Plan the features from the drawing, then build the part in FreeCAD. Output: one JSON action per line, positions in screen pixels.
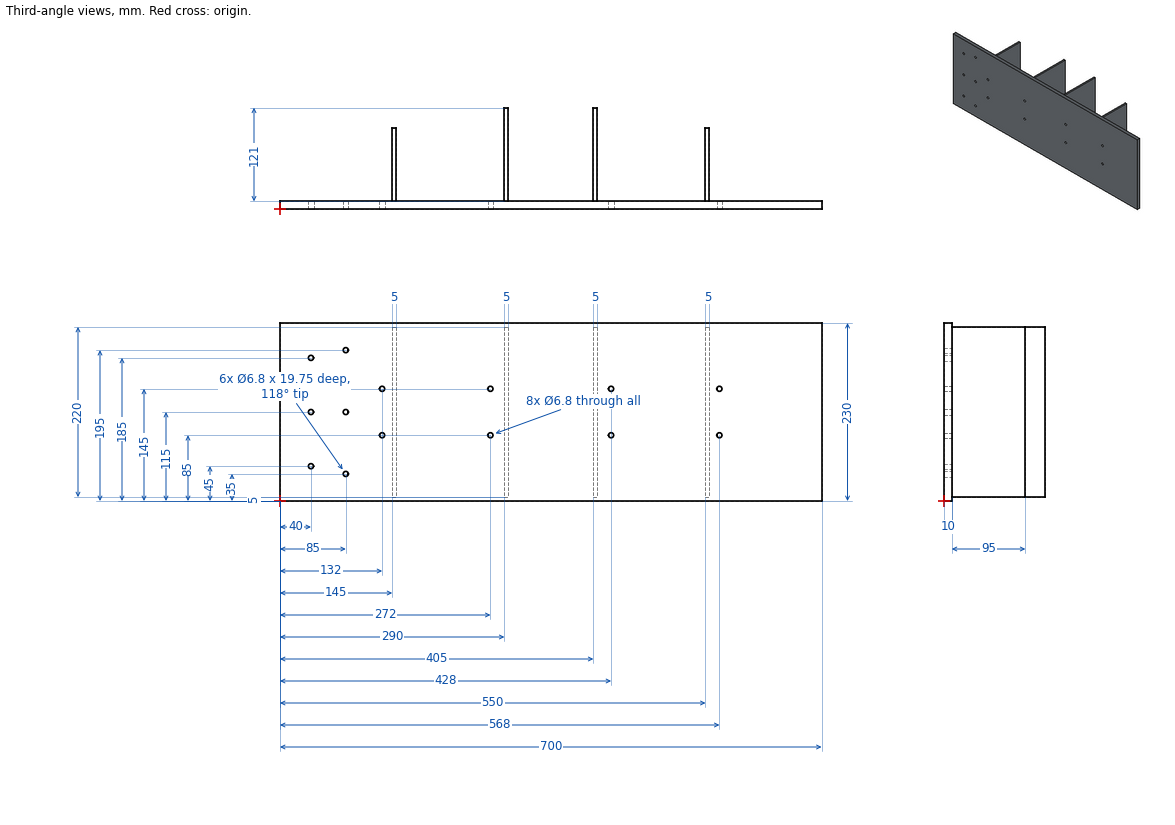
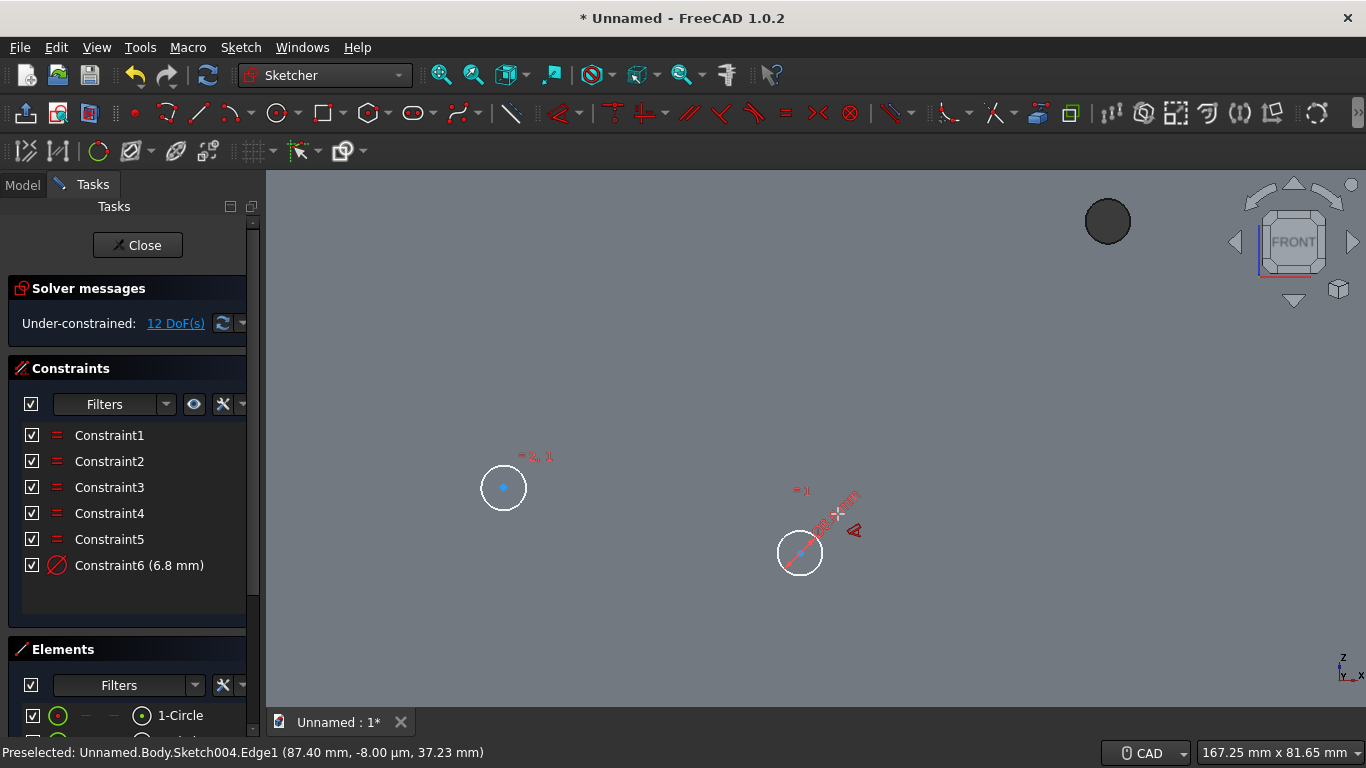
{"action": "scroll", "coordinate": [819, 540], "scroll_direction": "down", "scroll_amount": 7}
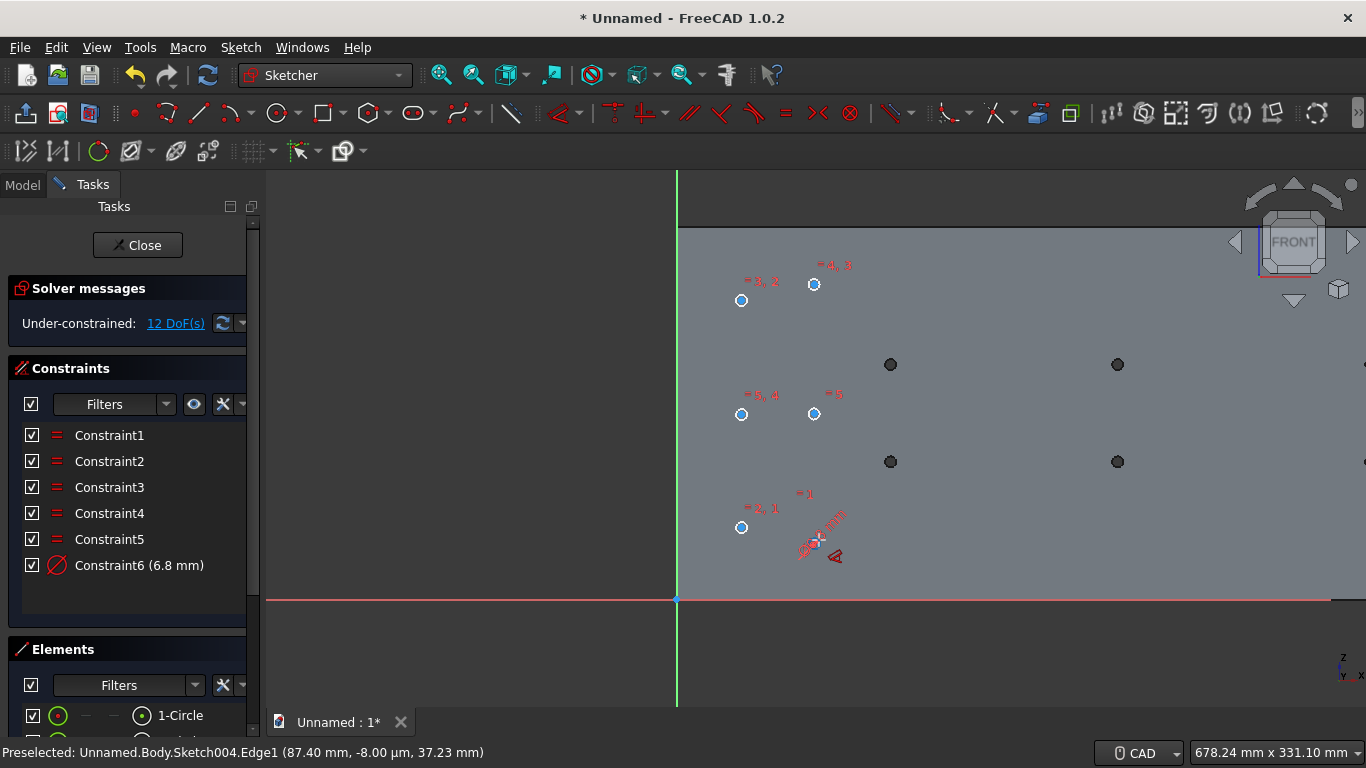
{"action": "left_click", "coordinate": [815, 544]}
{"action": "left_click", "coordinate": [746, 634]}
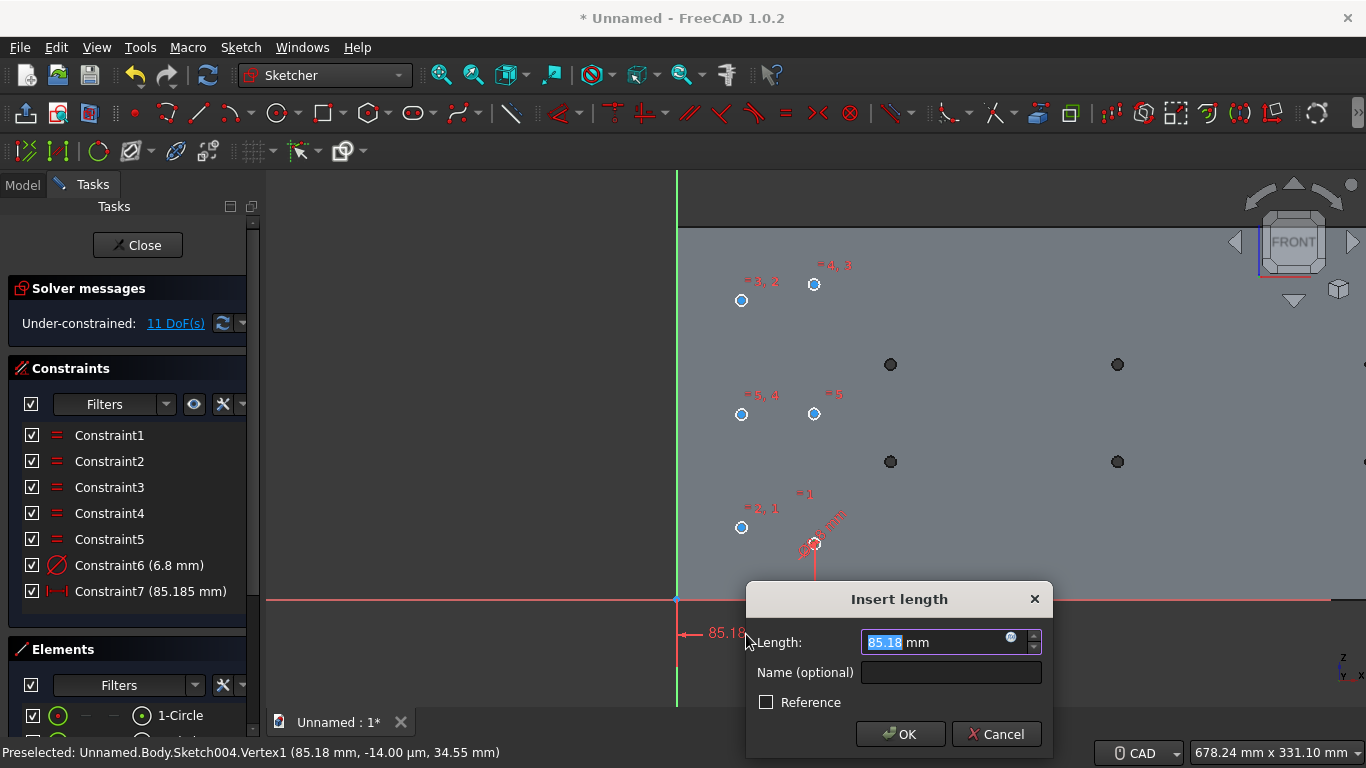
{"action": "type", "text": "85"}
{"action": "key", "text": "Return"}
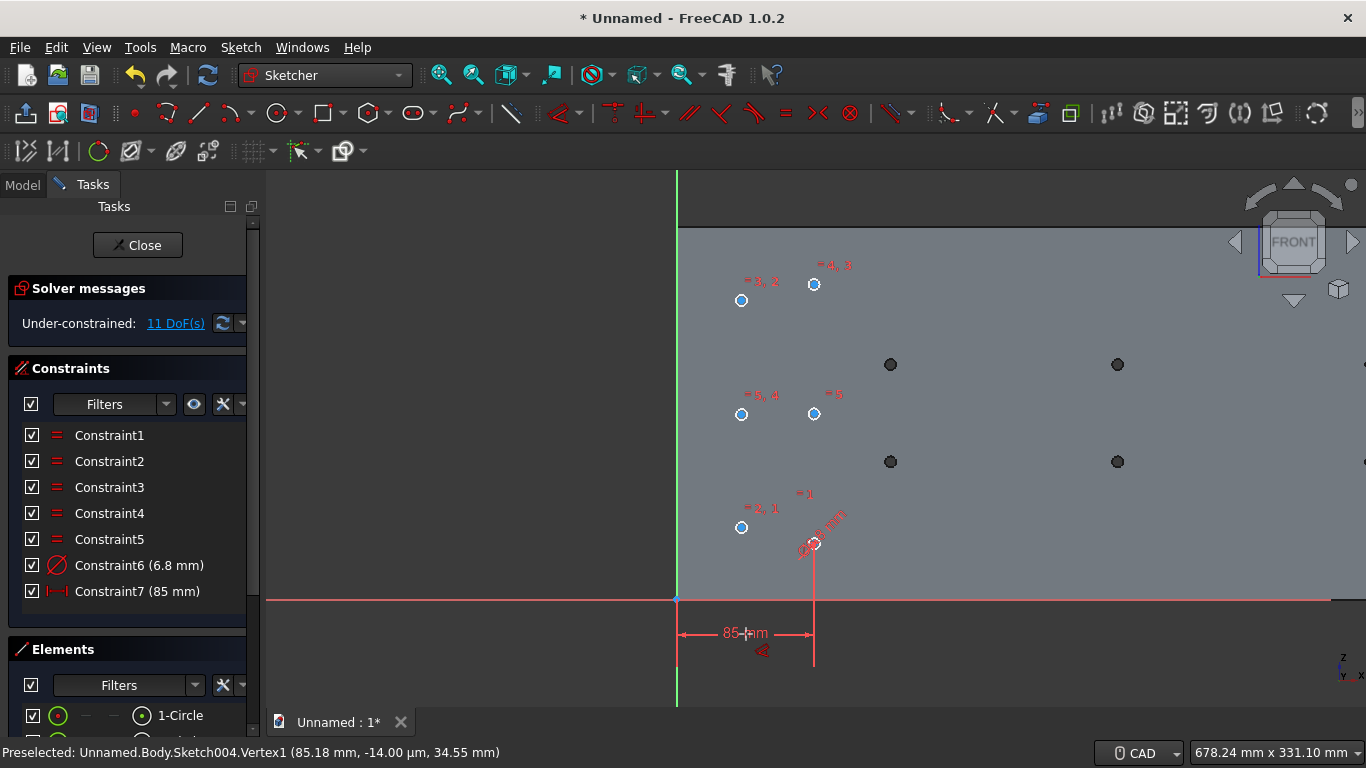
{"action": "left_click", "coordinate": [814, 544]}
{"action": "left_click", "coordinate": [643, 572]}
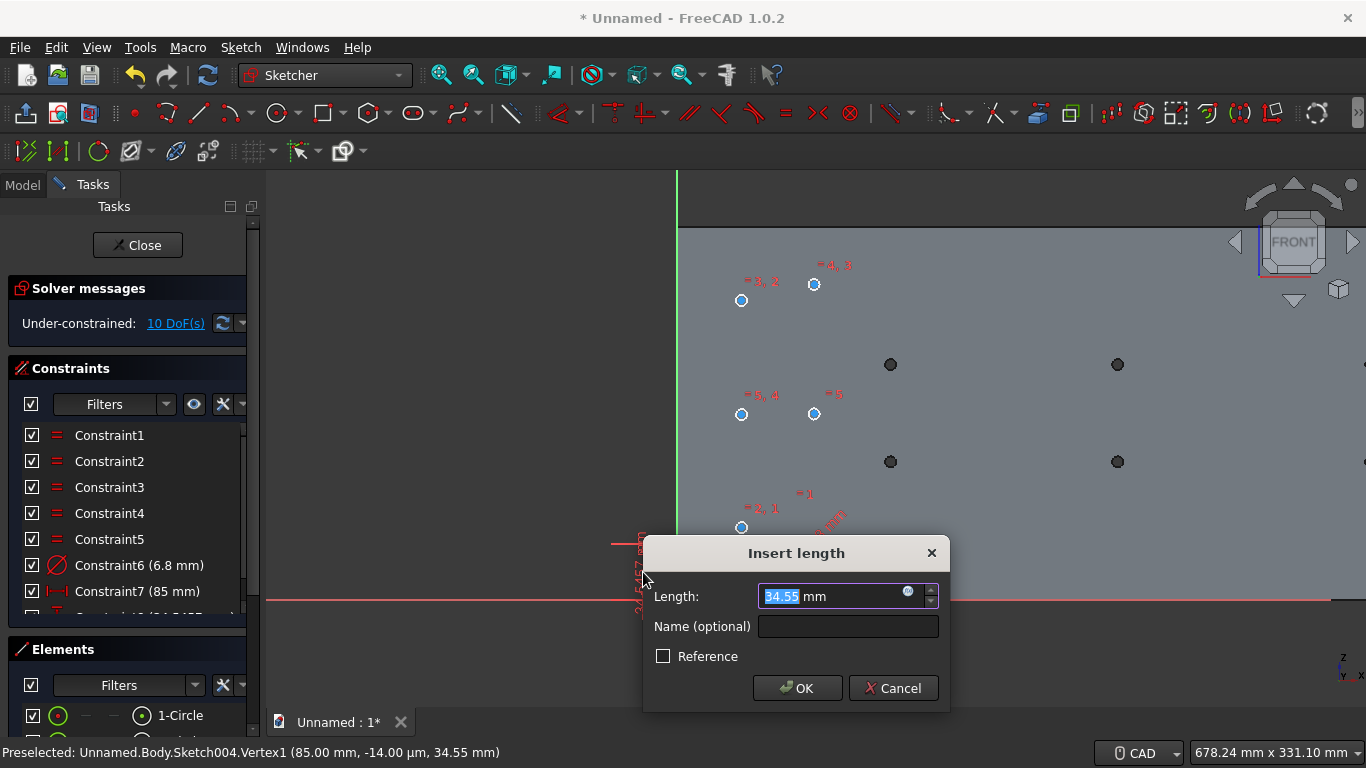
{"action": "type", "text": "35"}
{"action": "key", "text": "Return"}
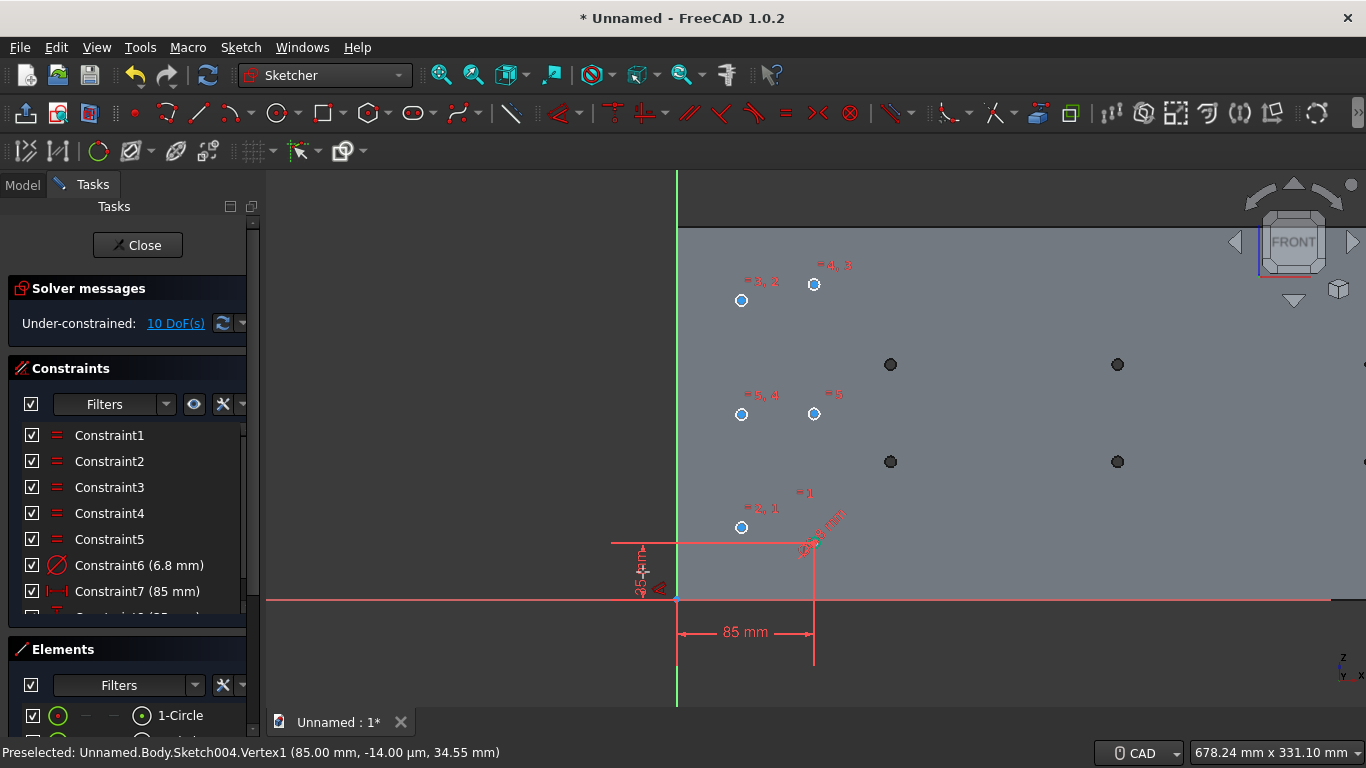
{"action": "left_click", "coordinate": [742, 528]}
{"action": "left_click", "coordinate": [709, 494]}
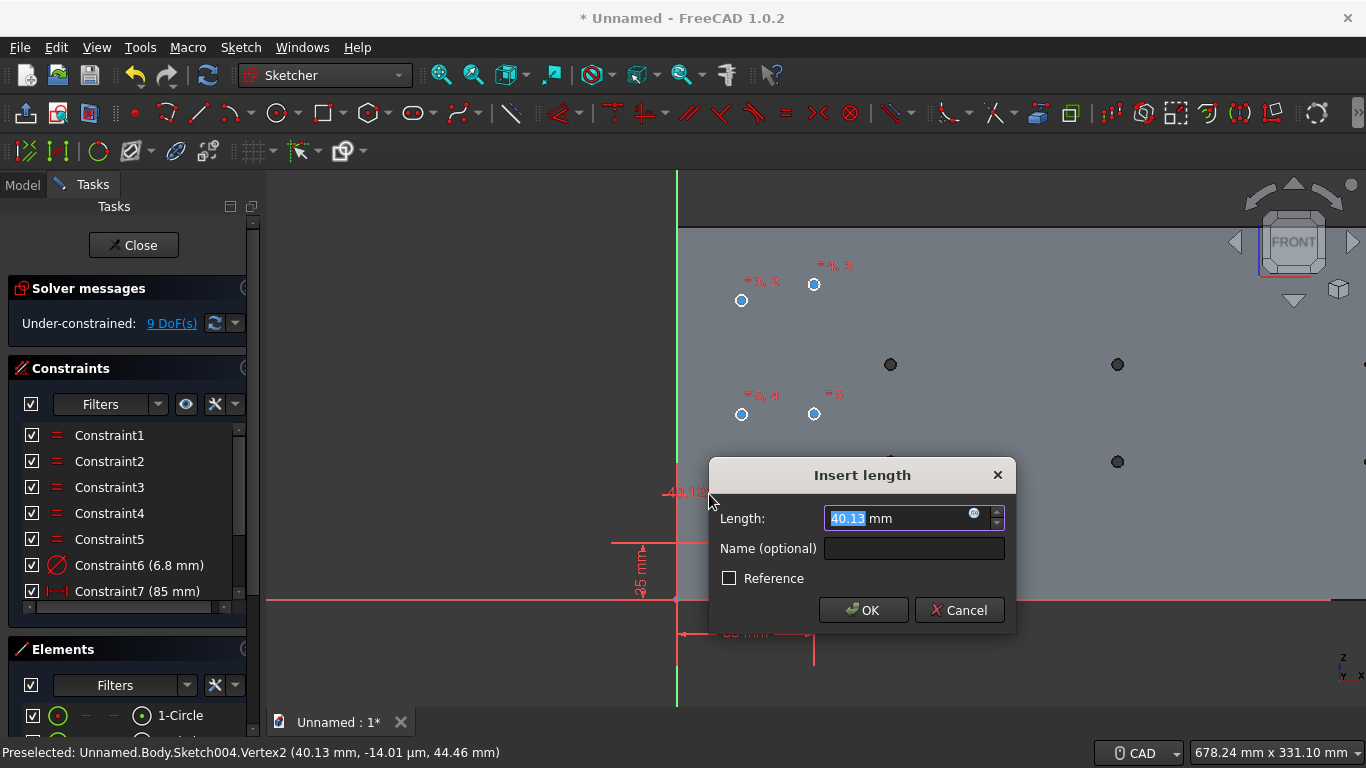
{"action": "type", "text": "40"}
{"action": "key", "text": "Return"}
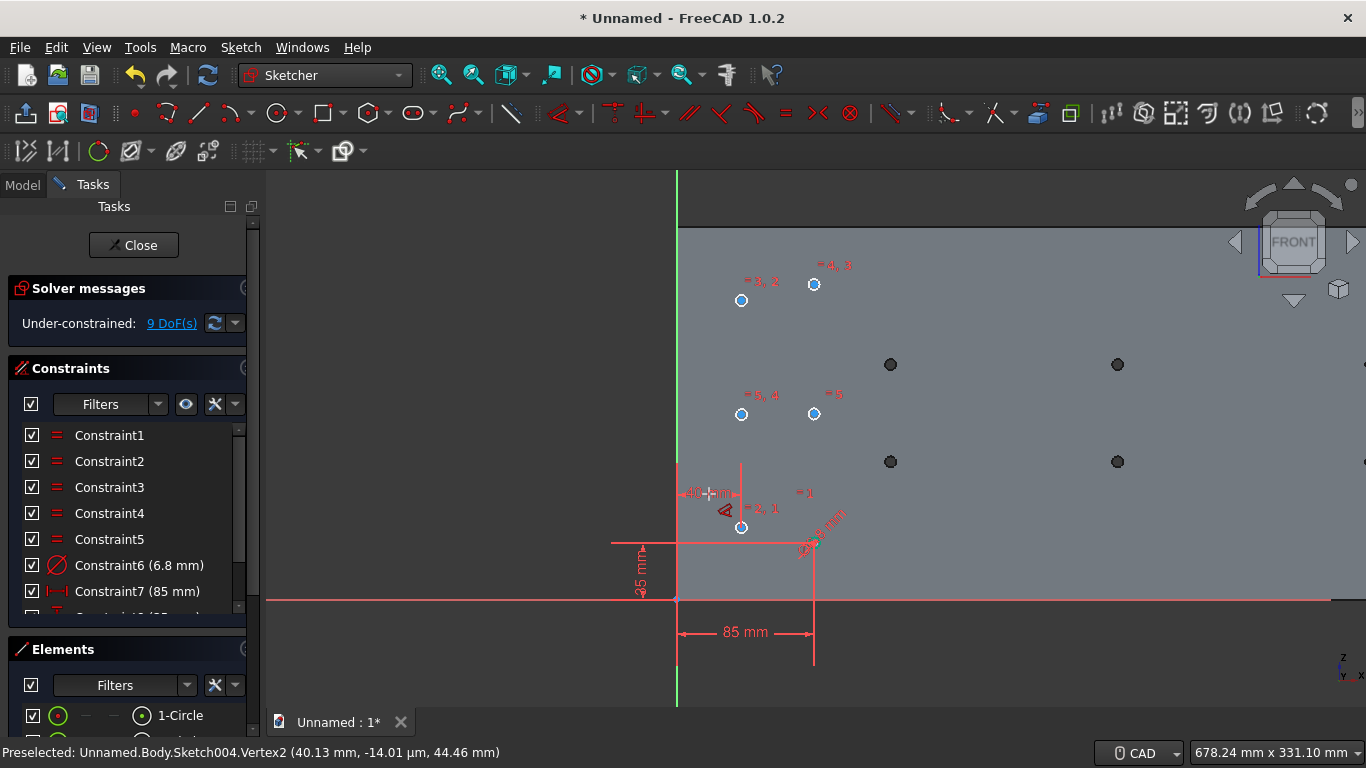
{"action": "left_click", "coordinate": [741, 528]}
{"action": "left_click", "coordinate": [643, 547]}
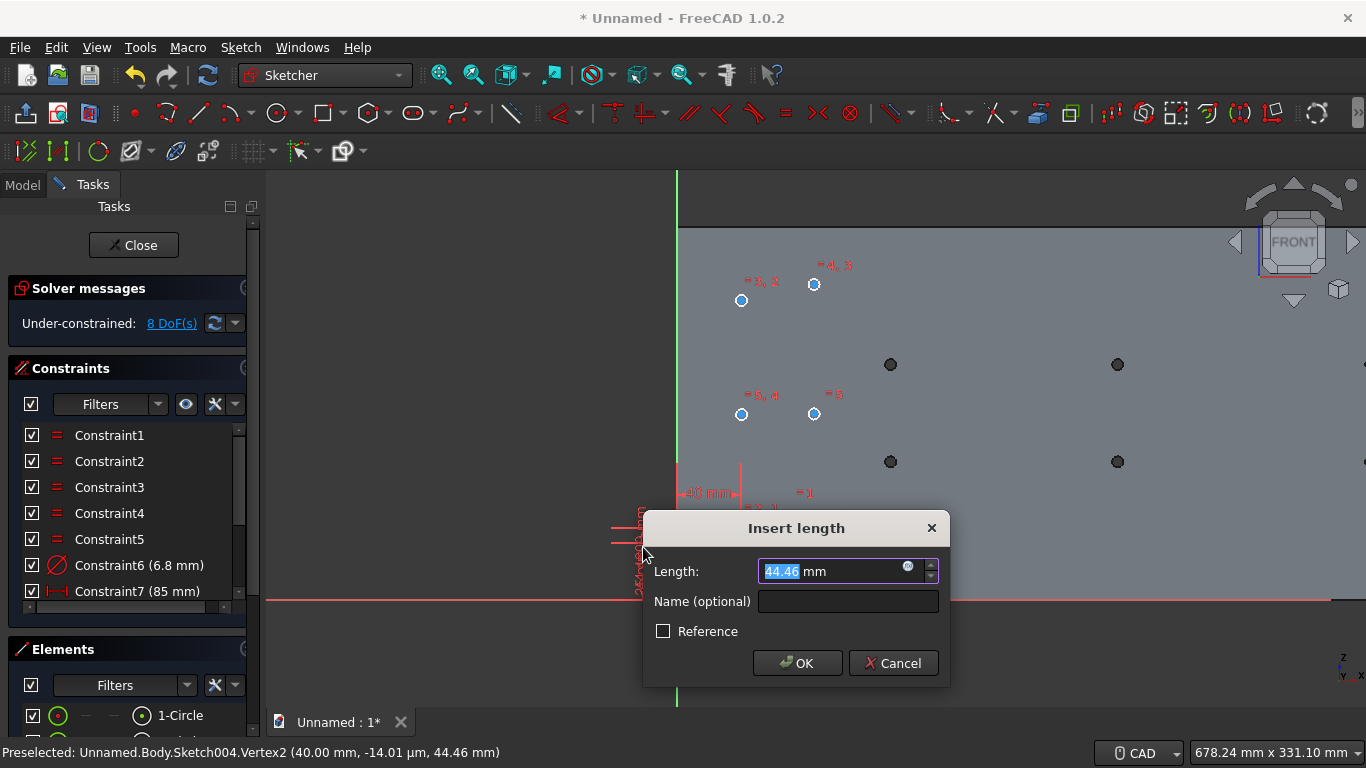
{"action": "type", "text": "45"}
{"action": "key", "text": "Return"}